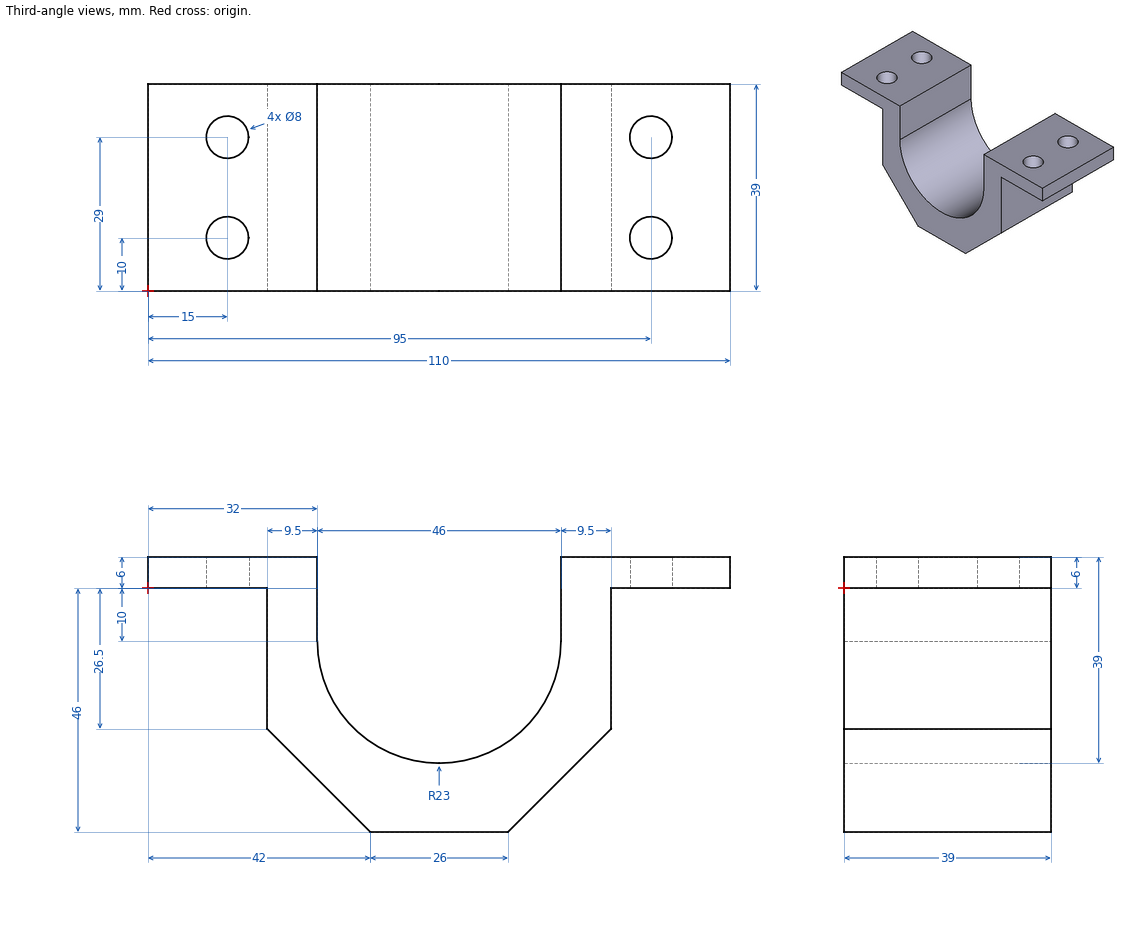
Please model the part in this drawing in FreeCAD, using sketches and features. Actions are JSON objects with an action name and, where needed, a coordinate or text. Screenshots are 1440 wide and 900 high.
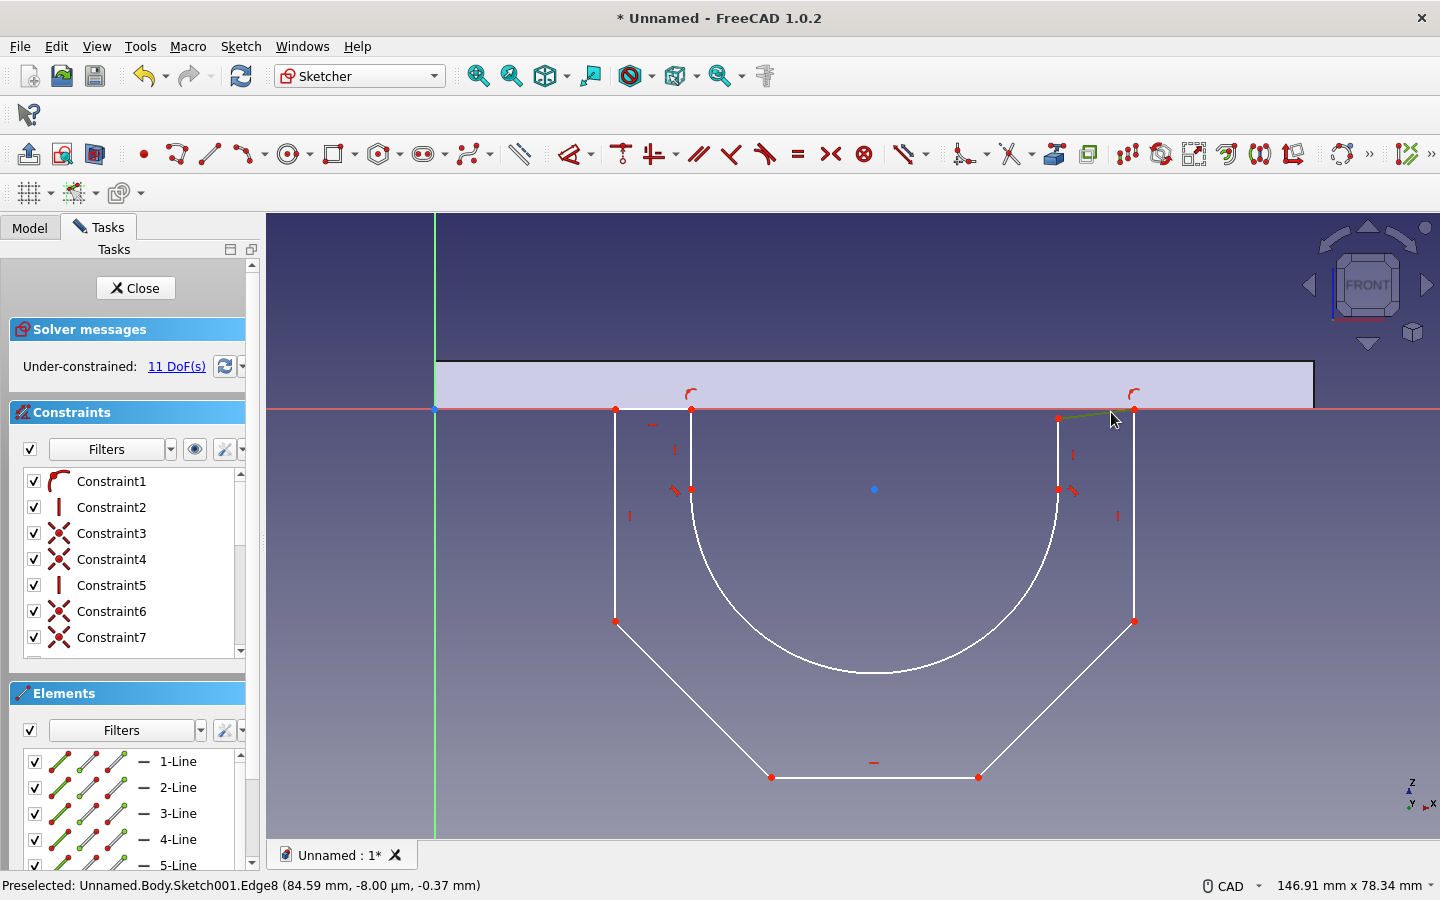
{"action": "key", "text": "h"}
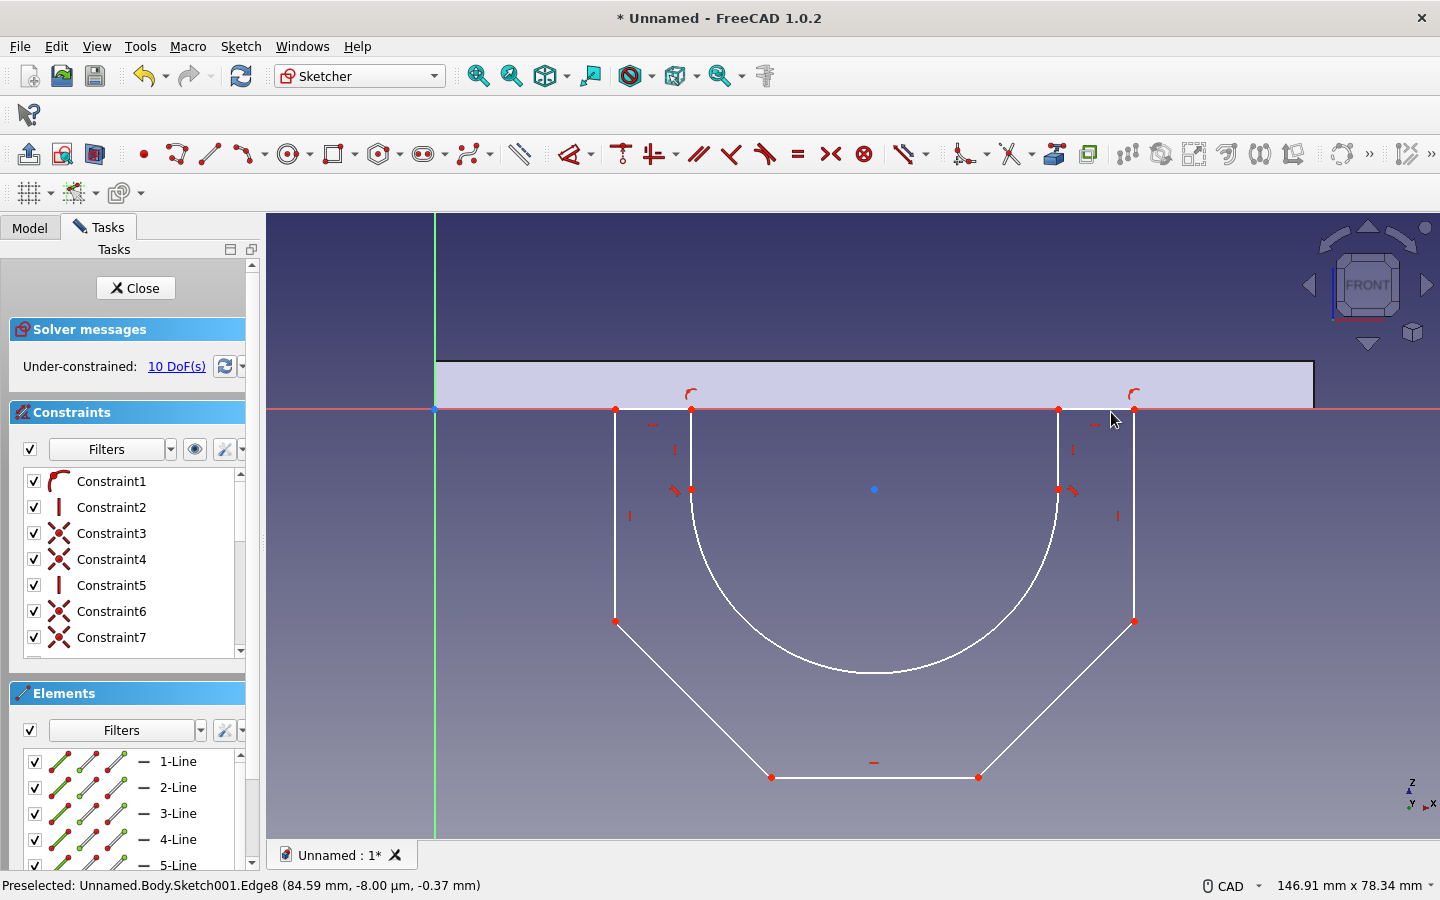
{"action": "key", "text": "d"}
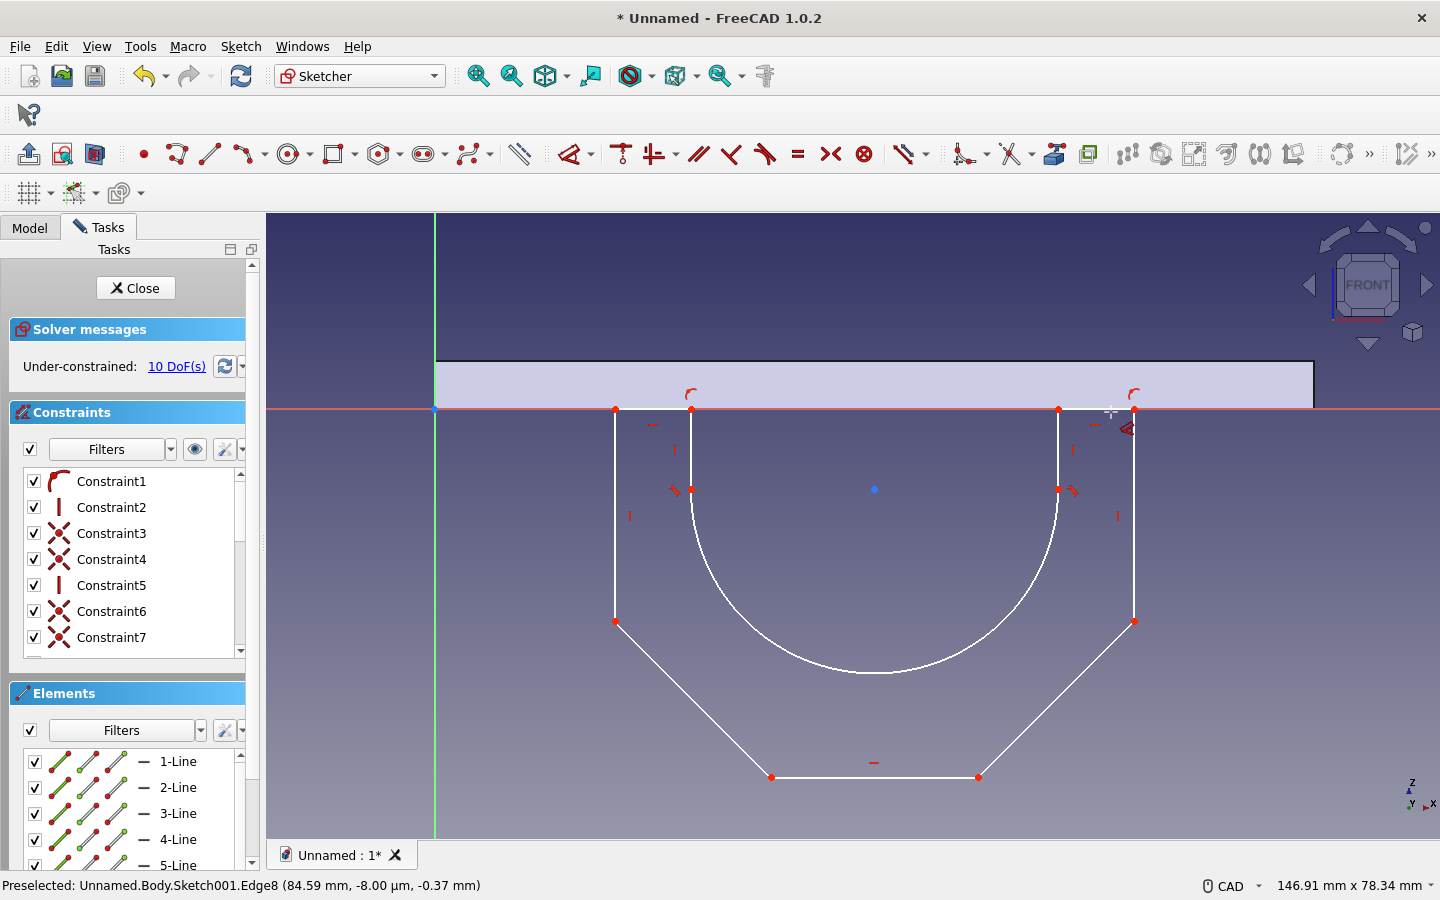
{"action": "left_click", "coordinate": [767, 638]}
{"action": "left_click", "coordinate": [748, 664]}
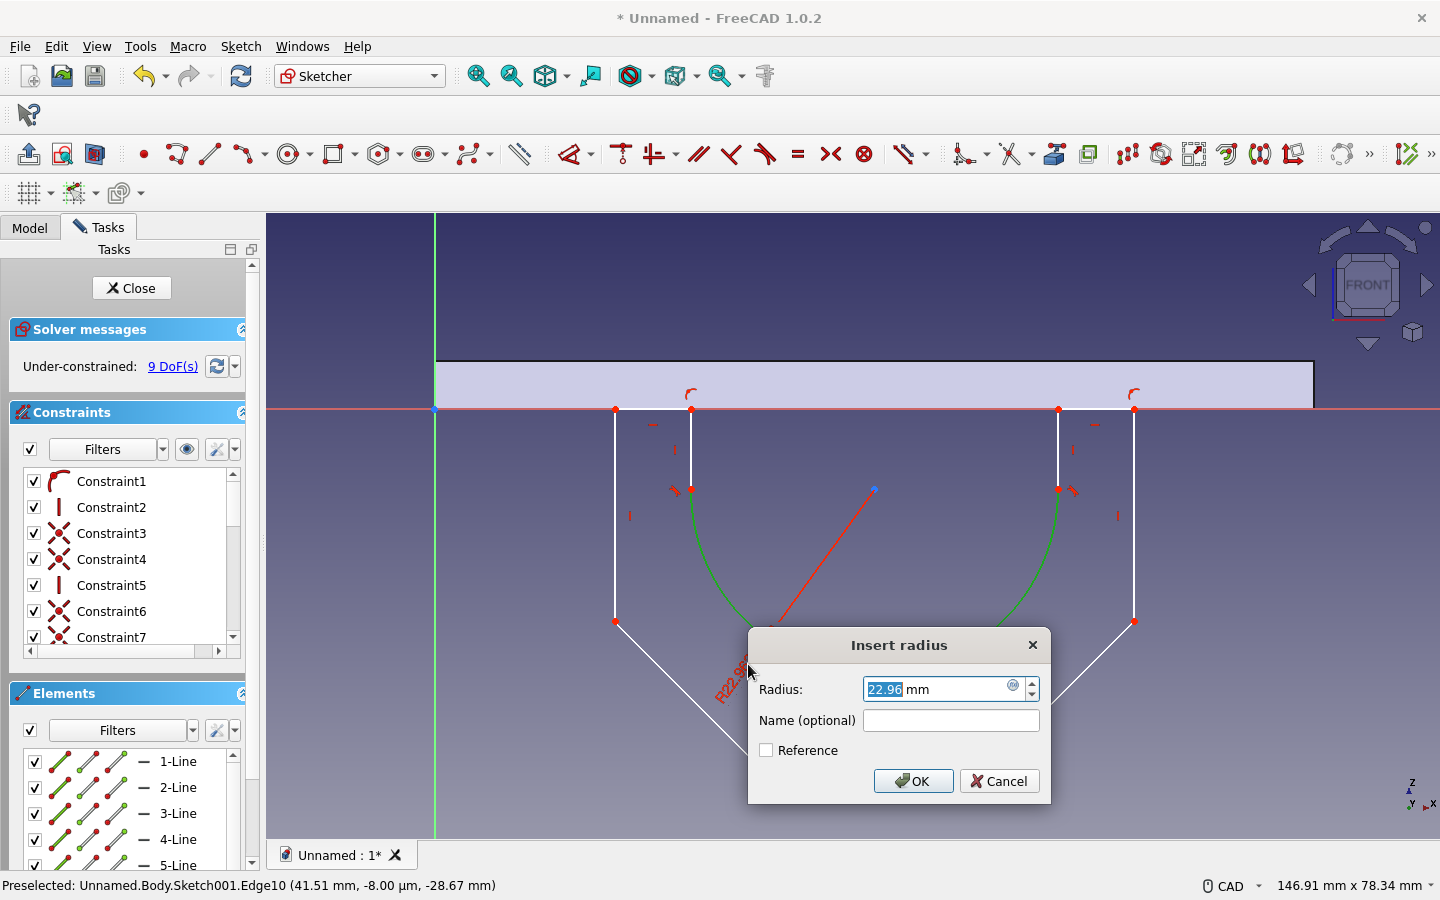
{"action": "type", "text": "23"}
{"action": "key", "text": "Return"}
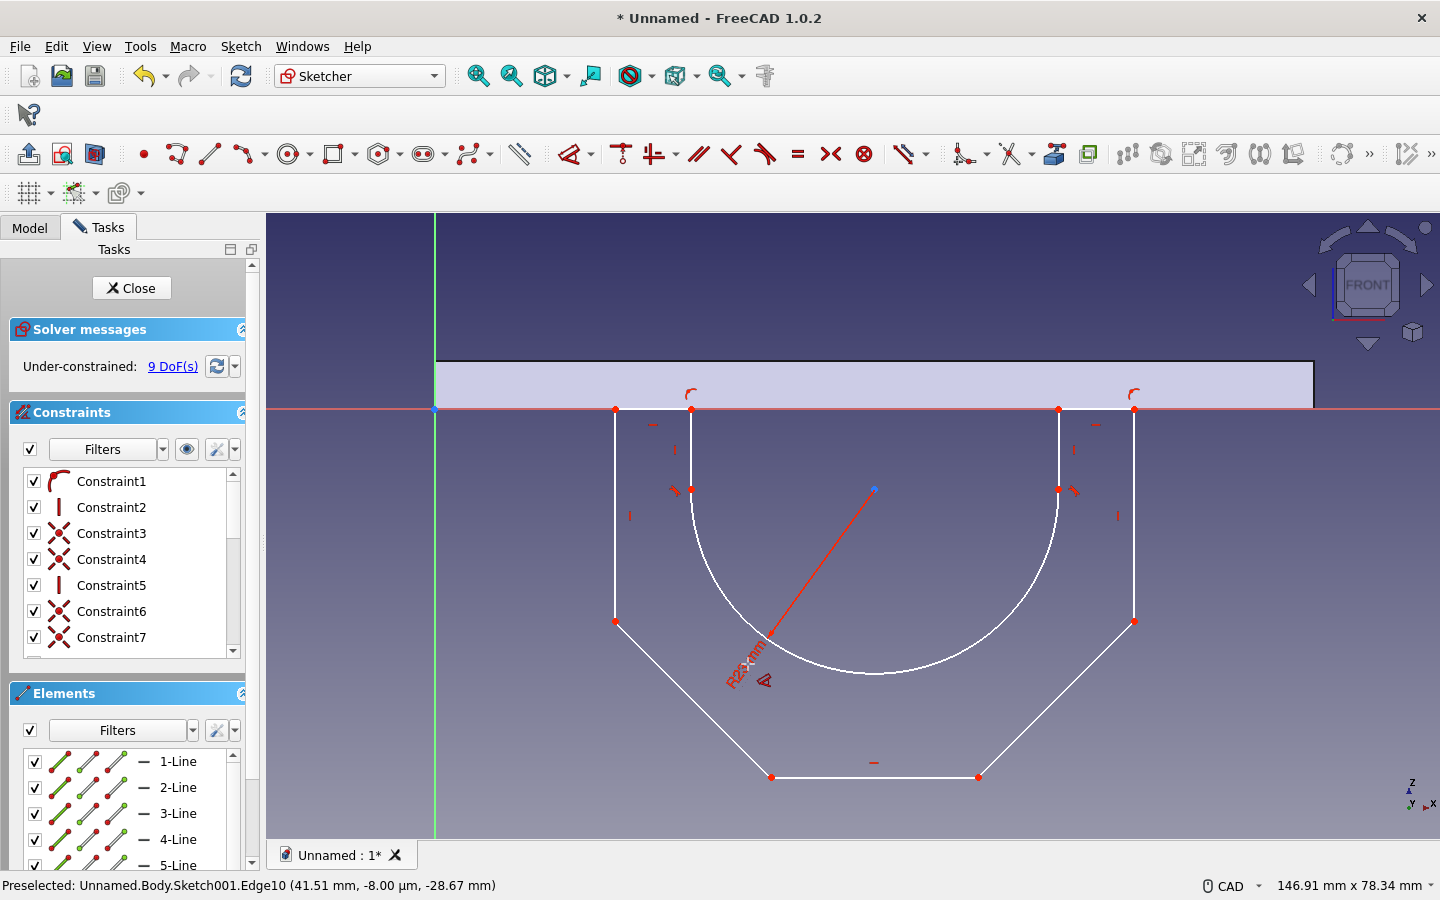
{"action": "left_click", "coordinate": [691, 466]}
{"action": "left_click", "coordinate": [657, 450]}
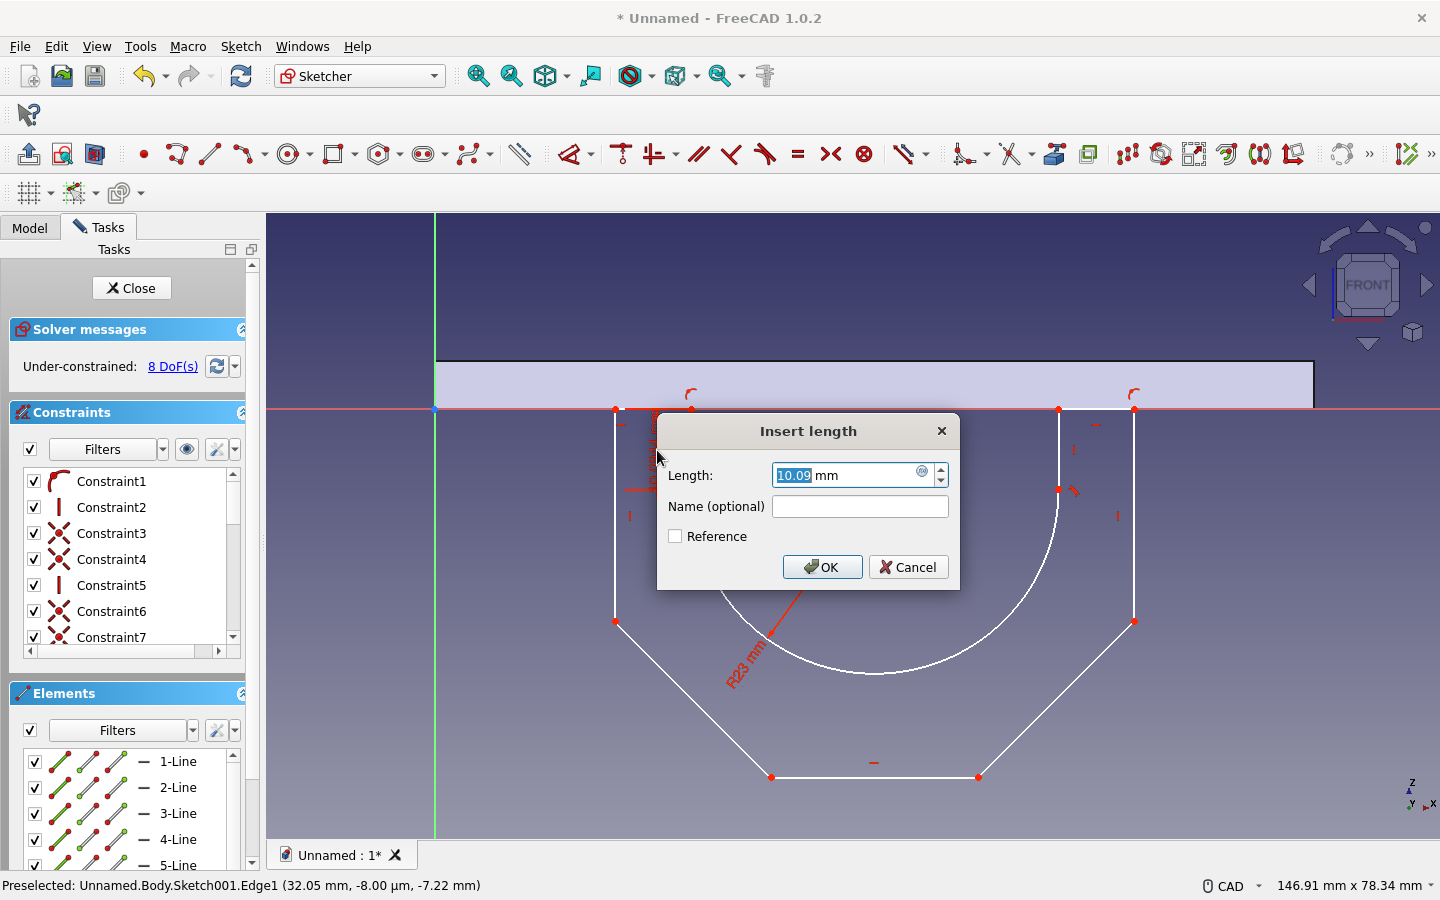
{"action": "type", "text": "10"}
{"action": "key", "text": "Return"}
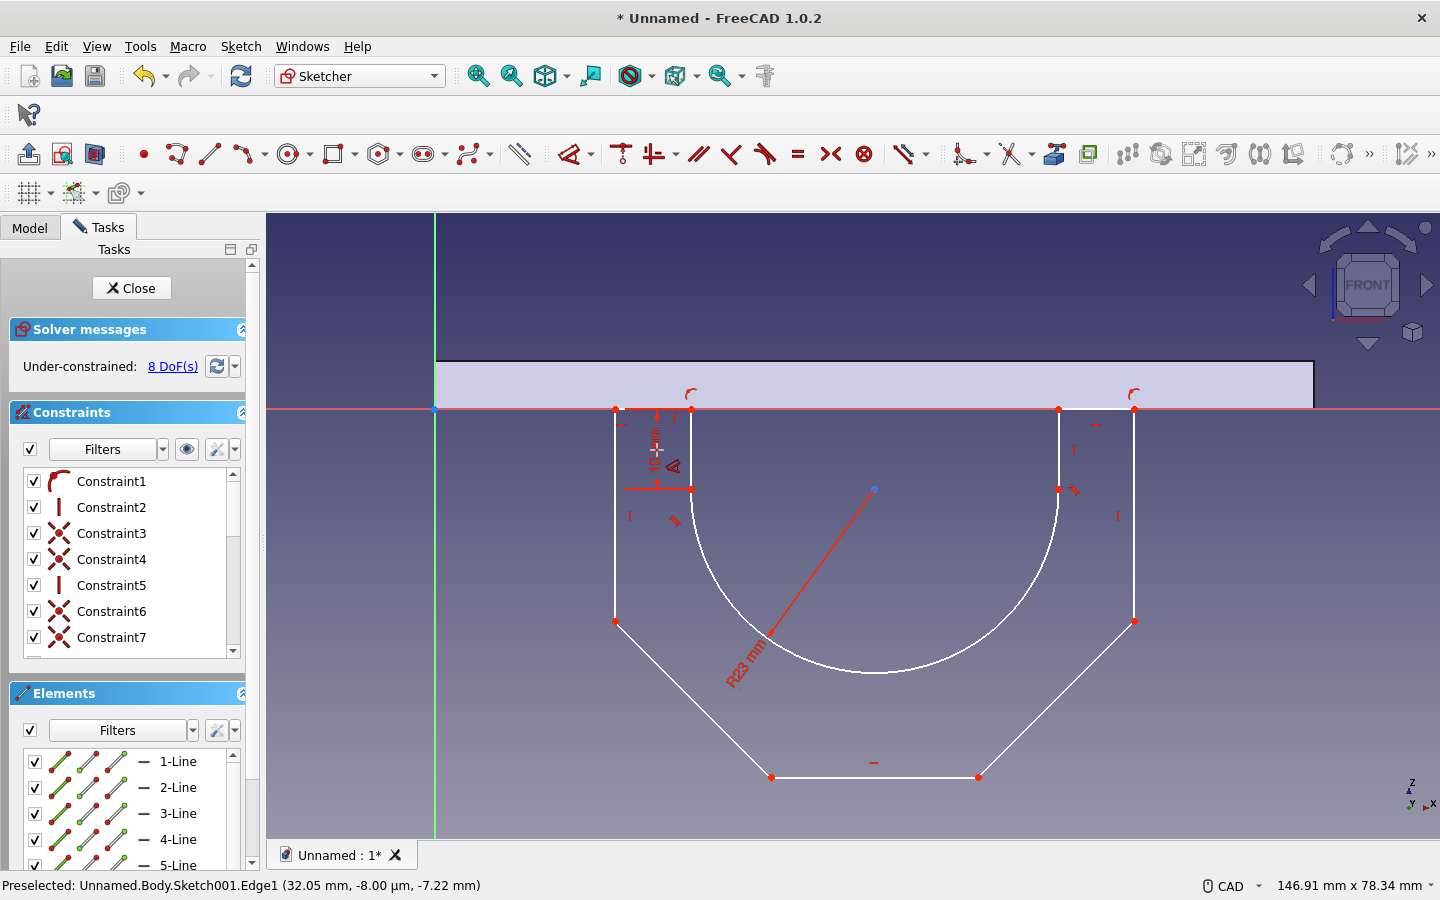
{"action": "left_click", "coordinate": [833, 778]}
{"action": "left_click", "coordinate": [874, 744]}